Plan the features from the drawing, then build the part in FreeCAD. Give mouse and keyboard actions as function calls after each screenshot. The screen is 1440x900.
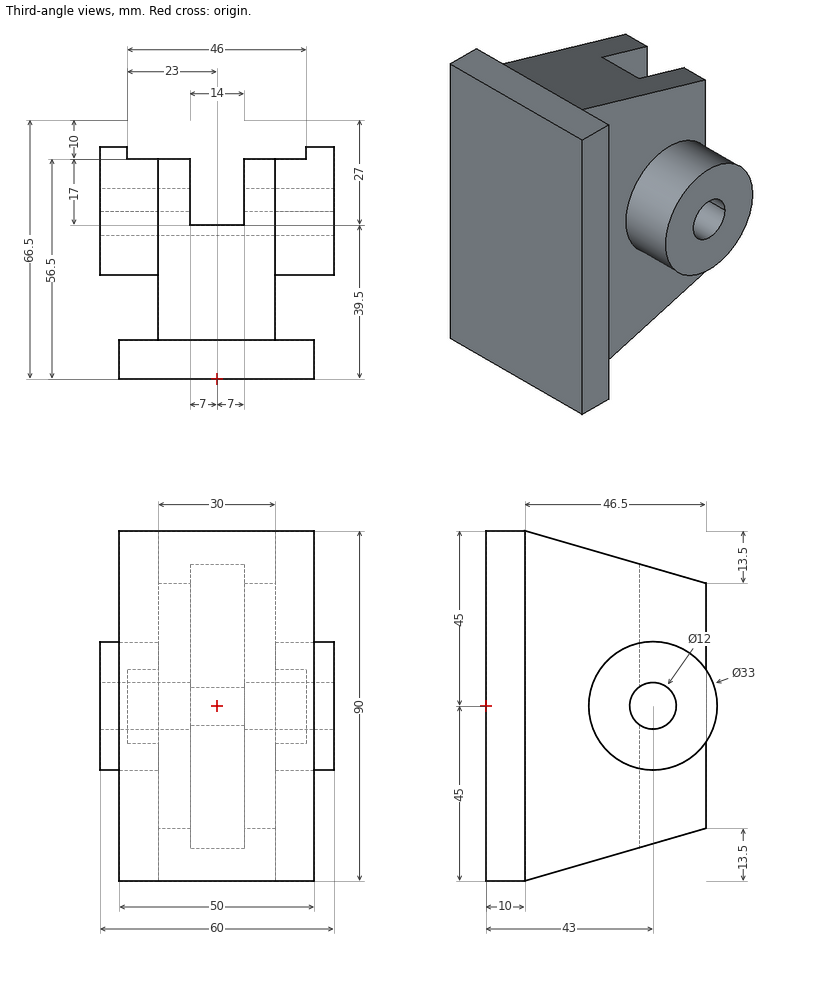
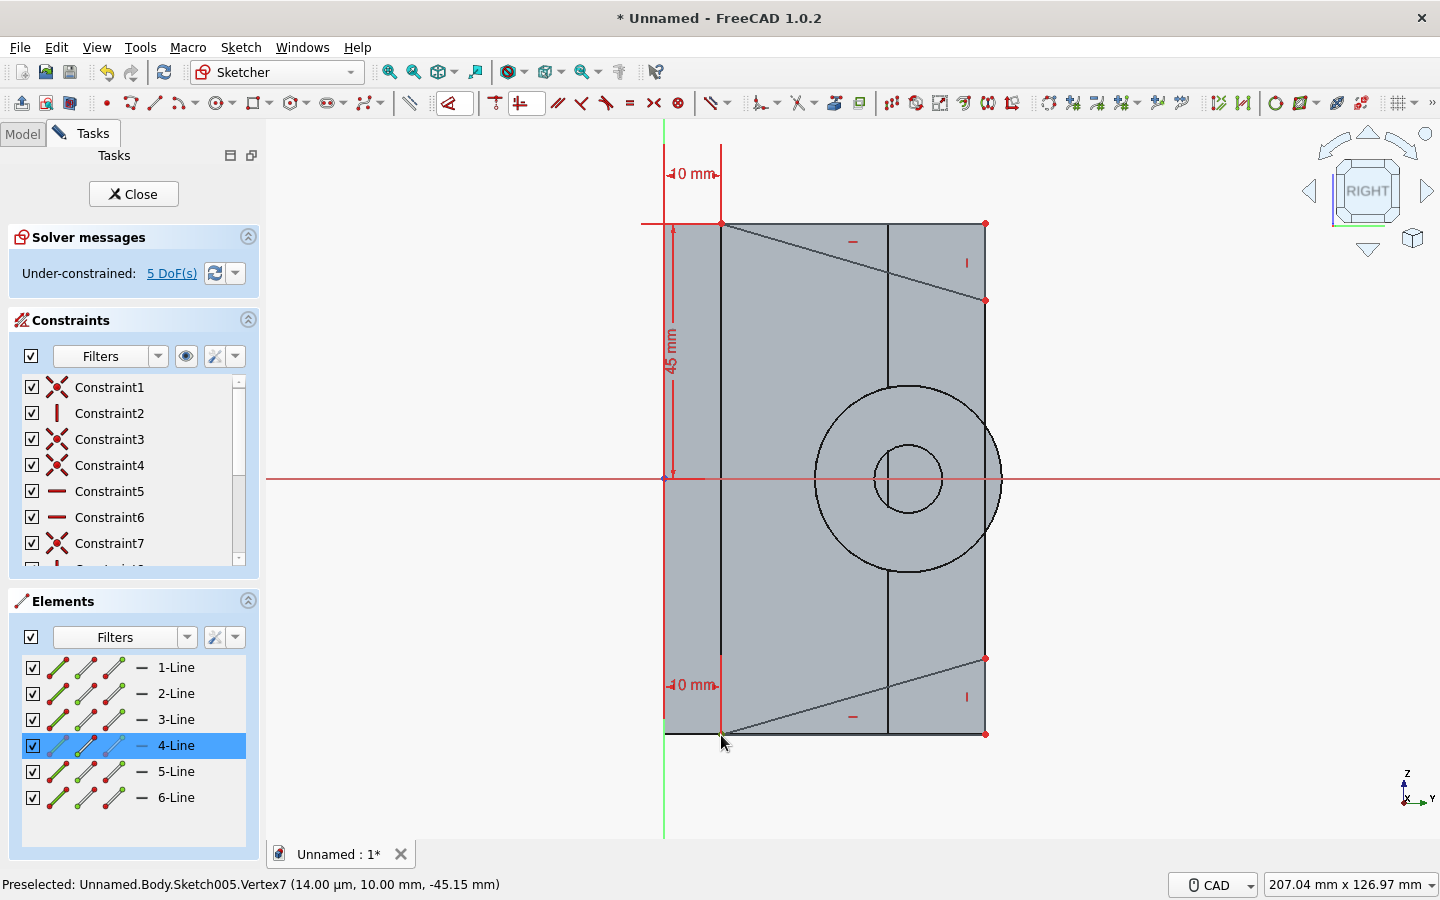
click(468, 104)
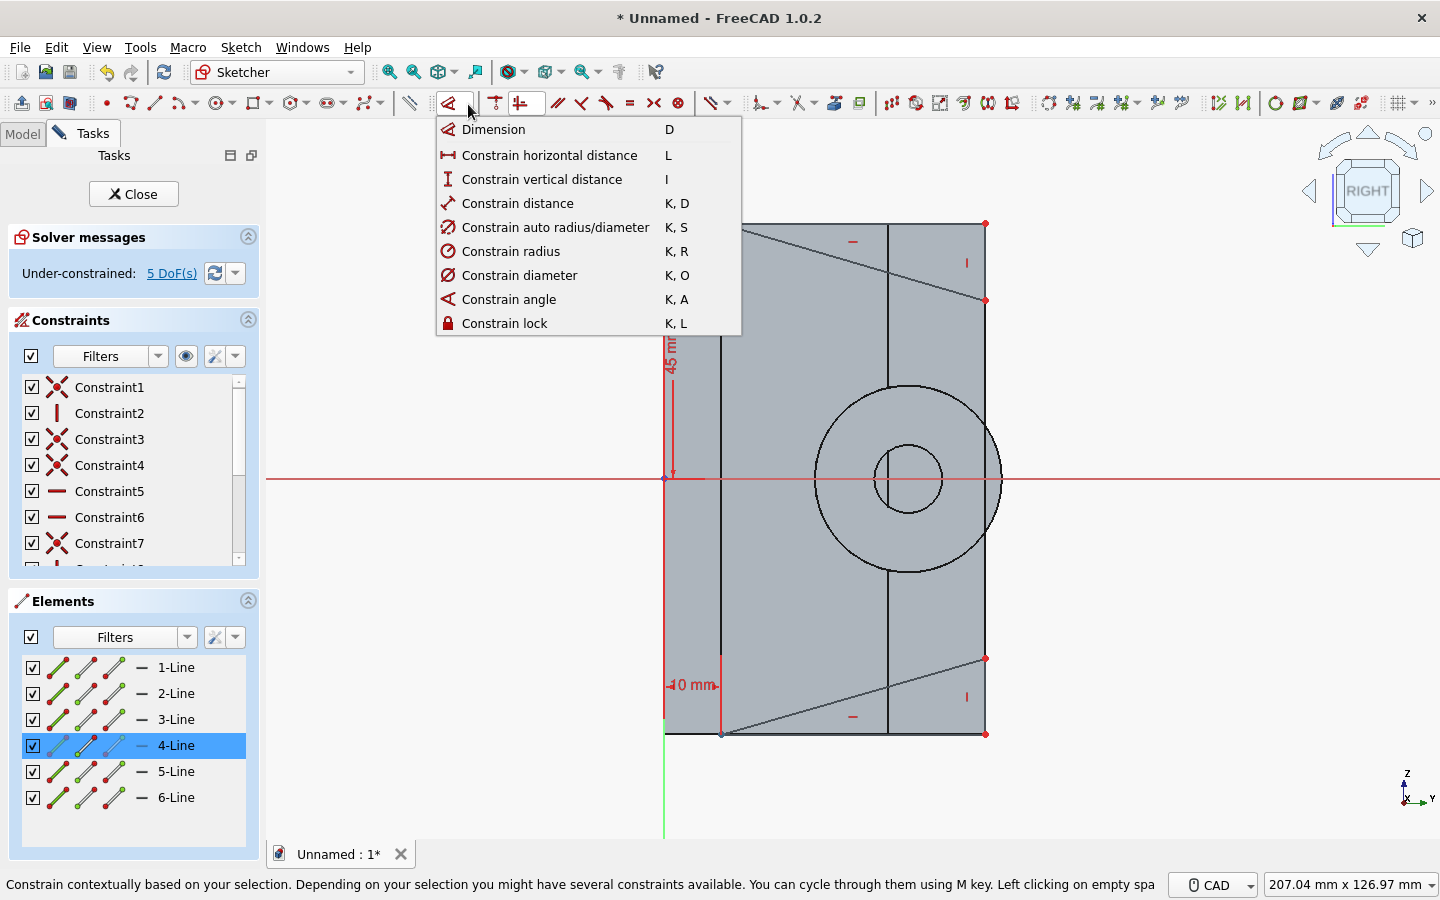
click(589, 179)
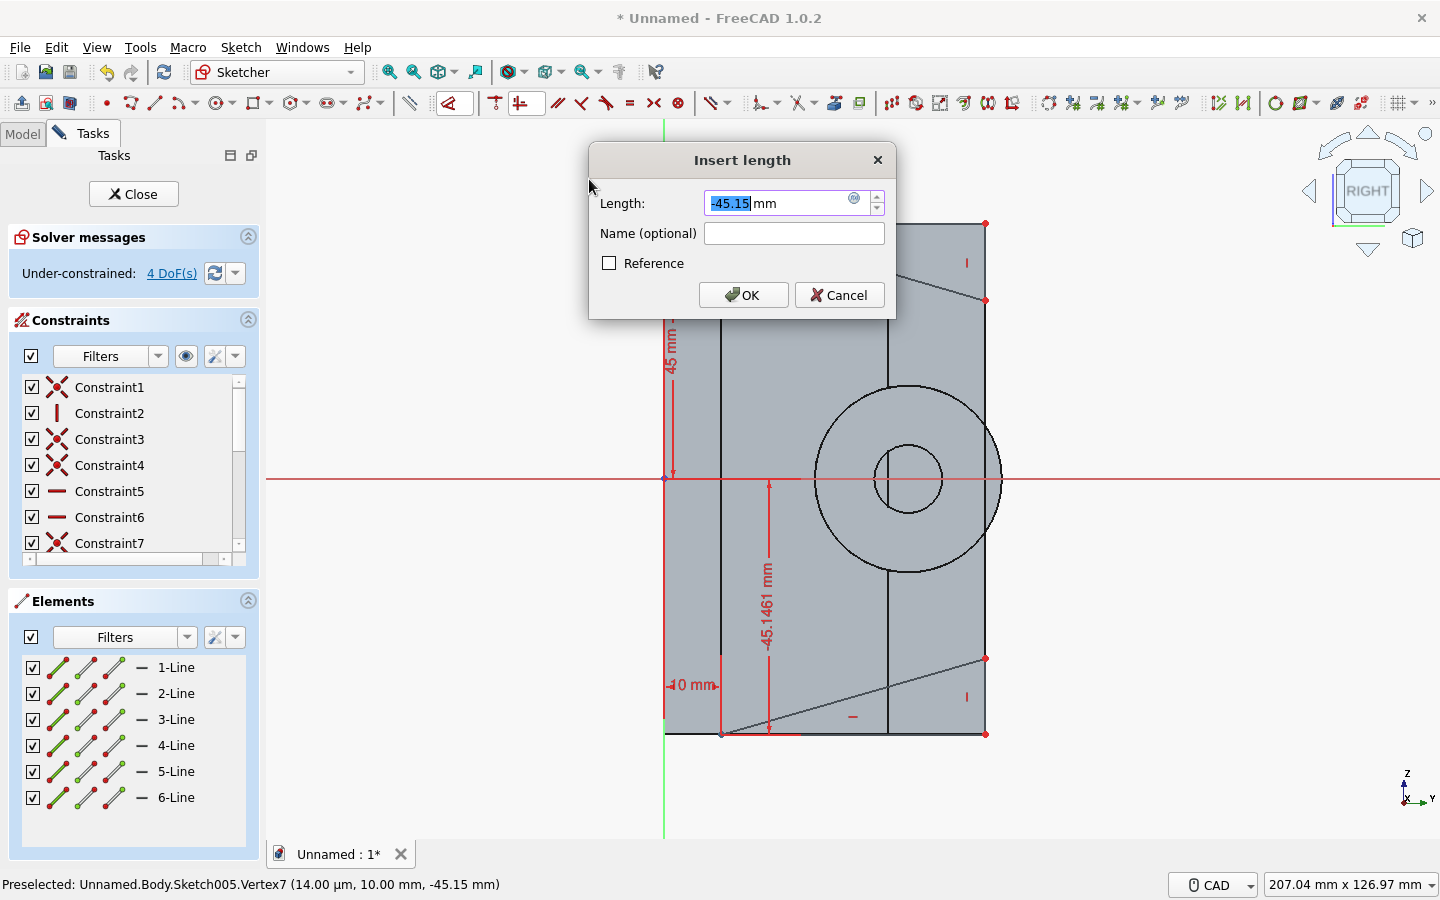
text(-45)
key(Return)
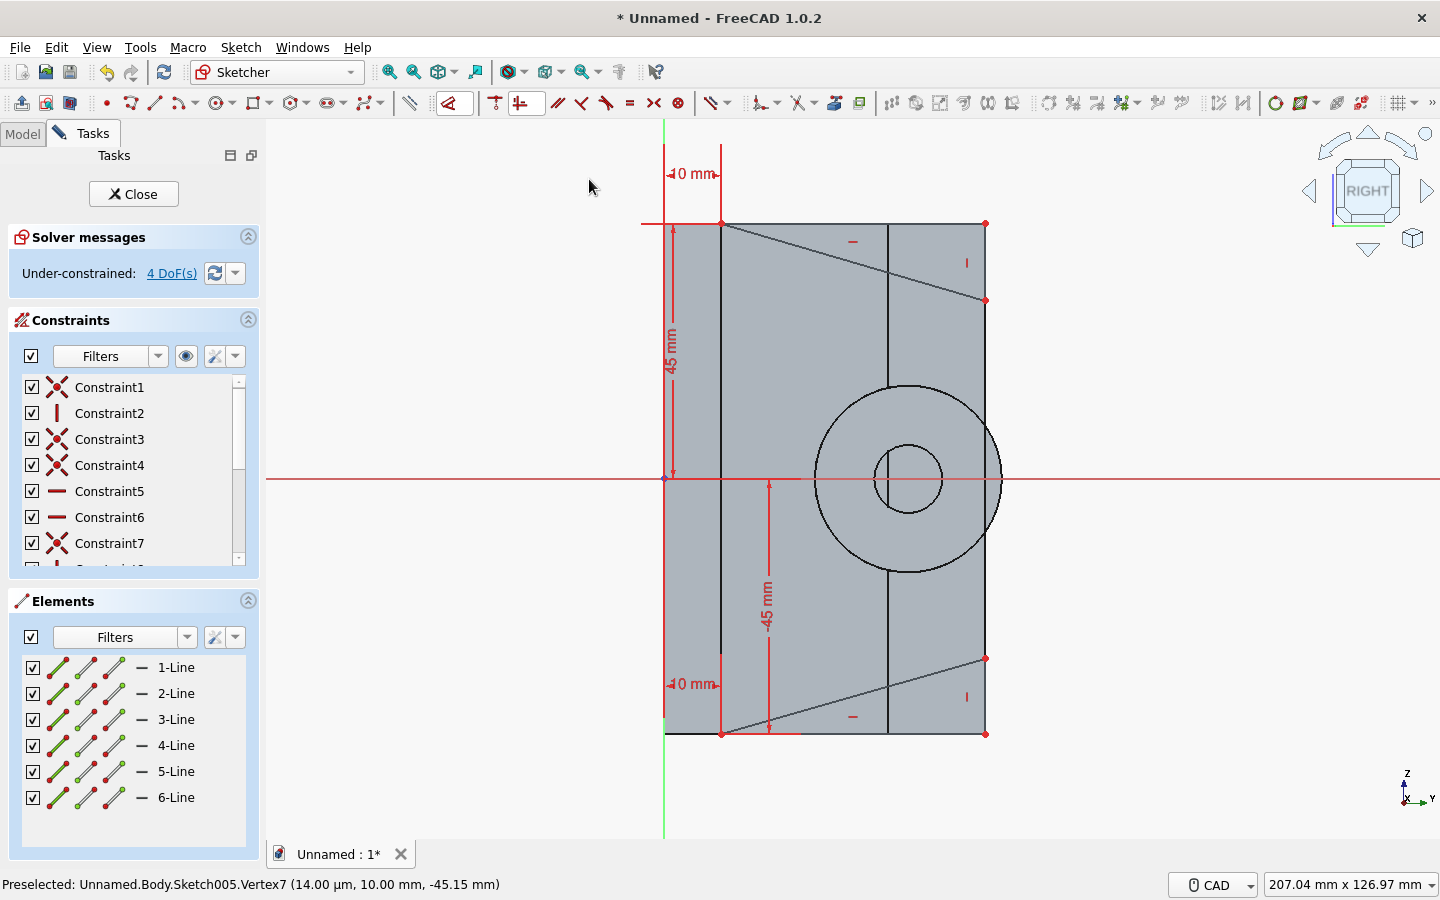
click(985, 278)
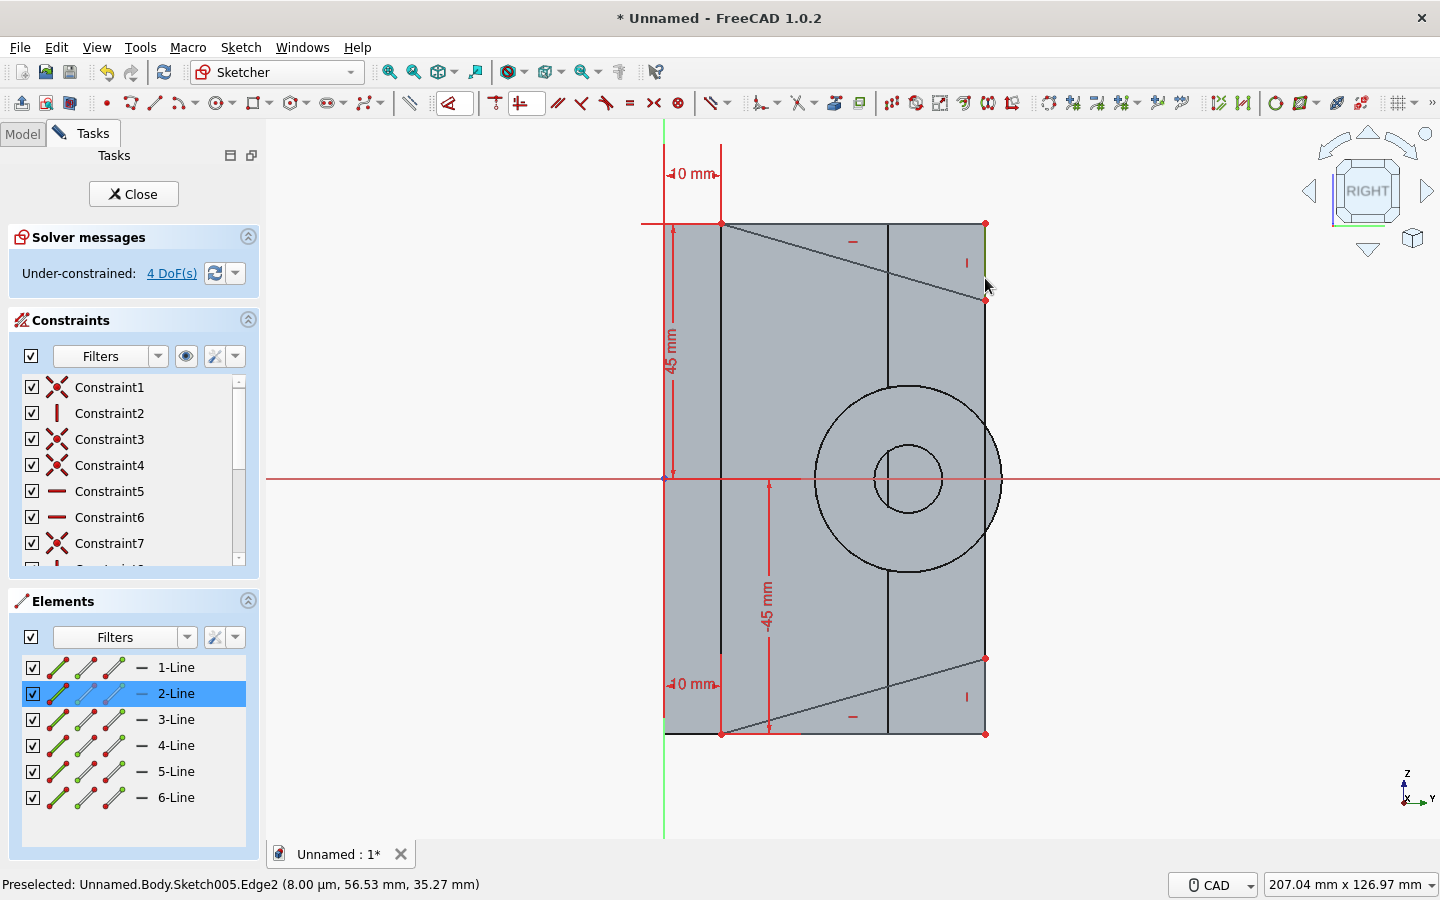
click(468, 104)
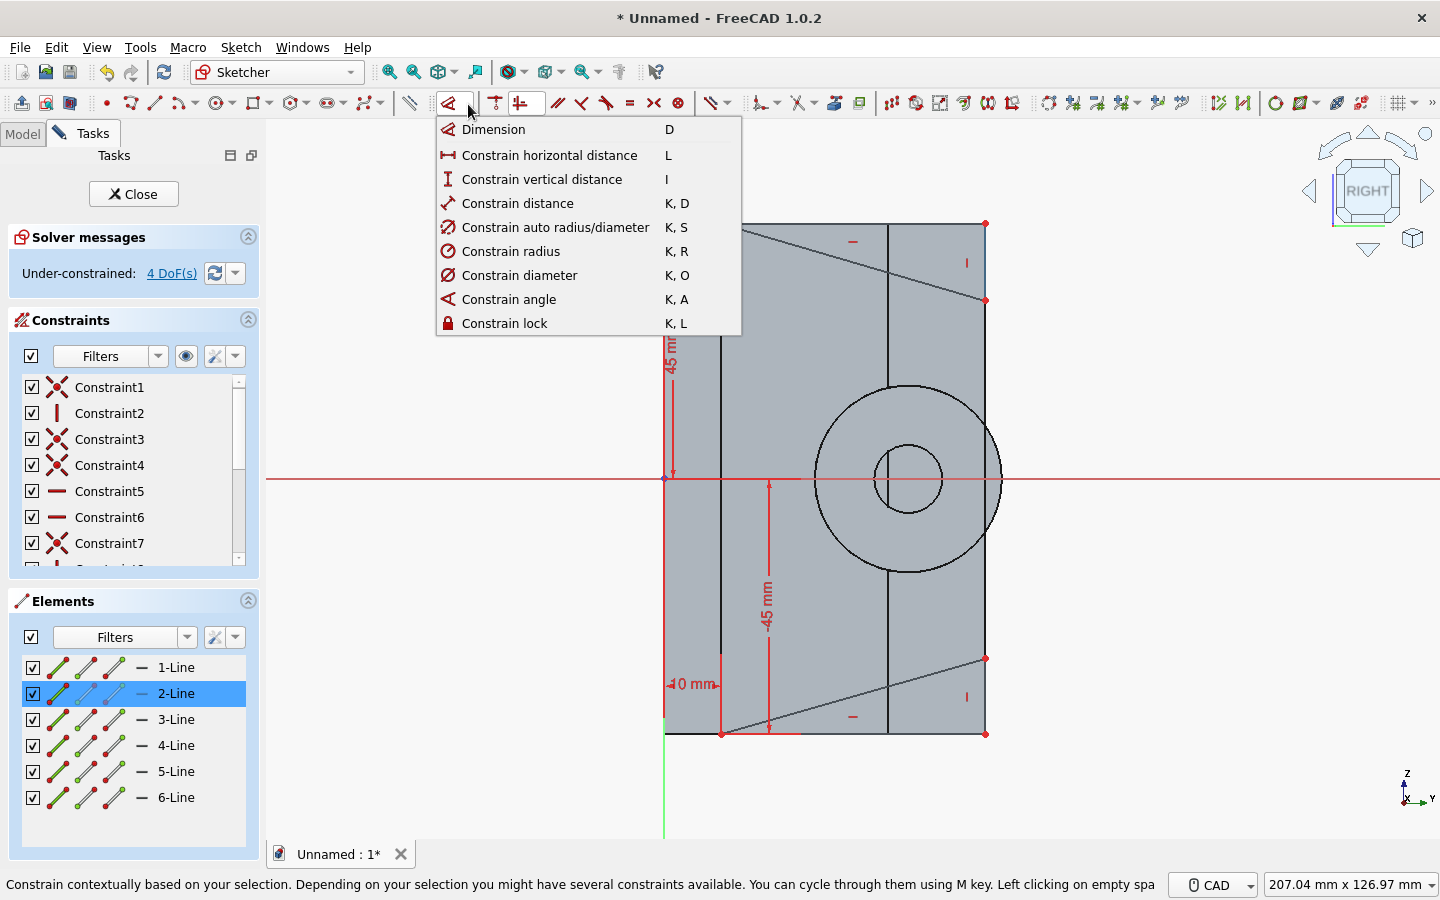
click(589, 179)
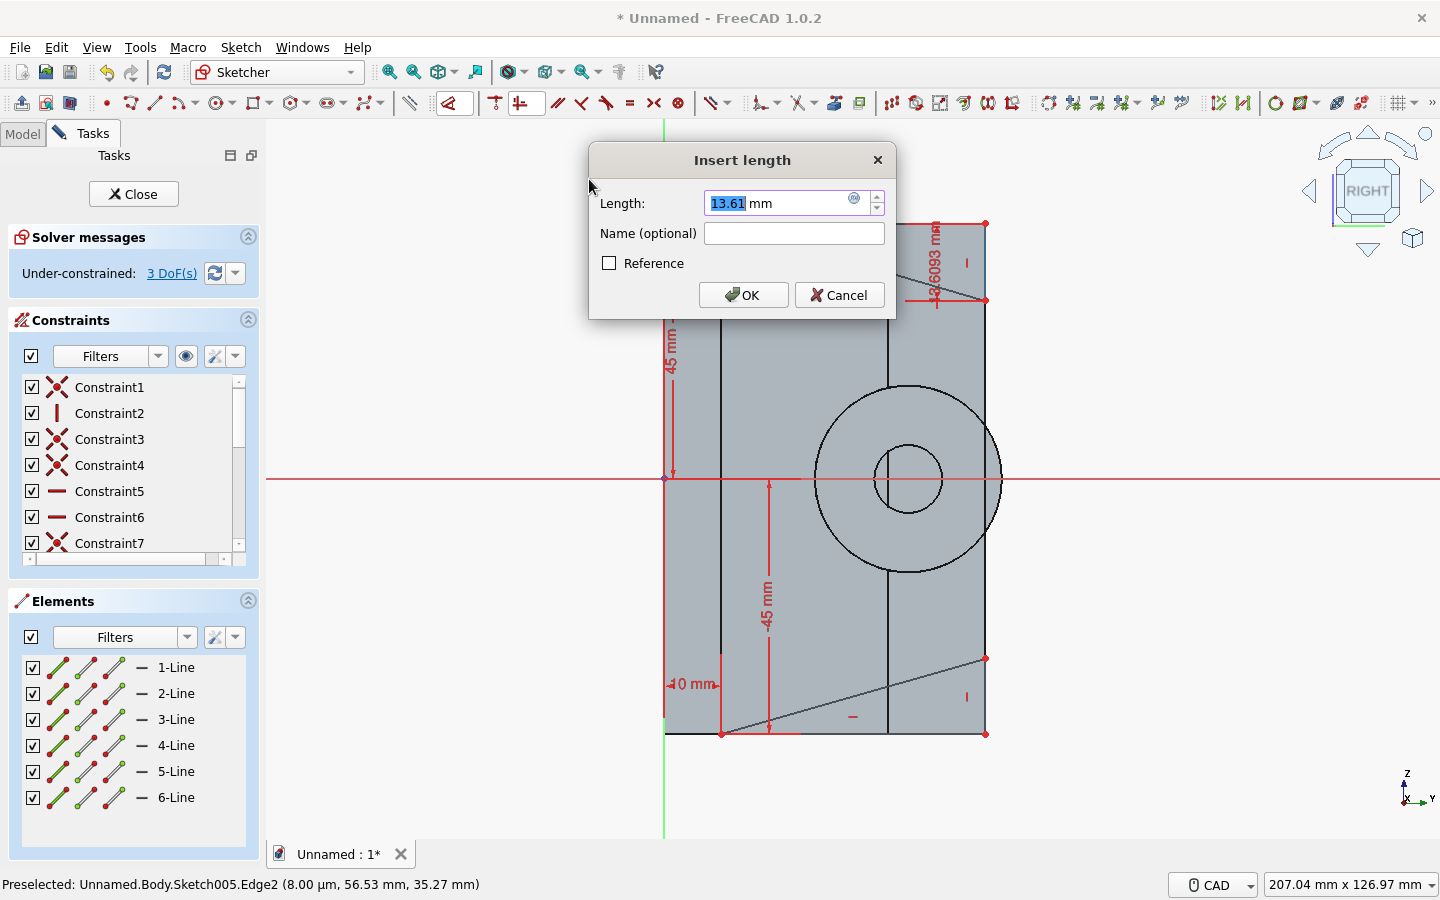
text(13.5)
key(Return)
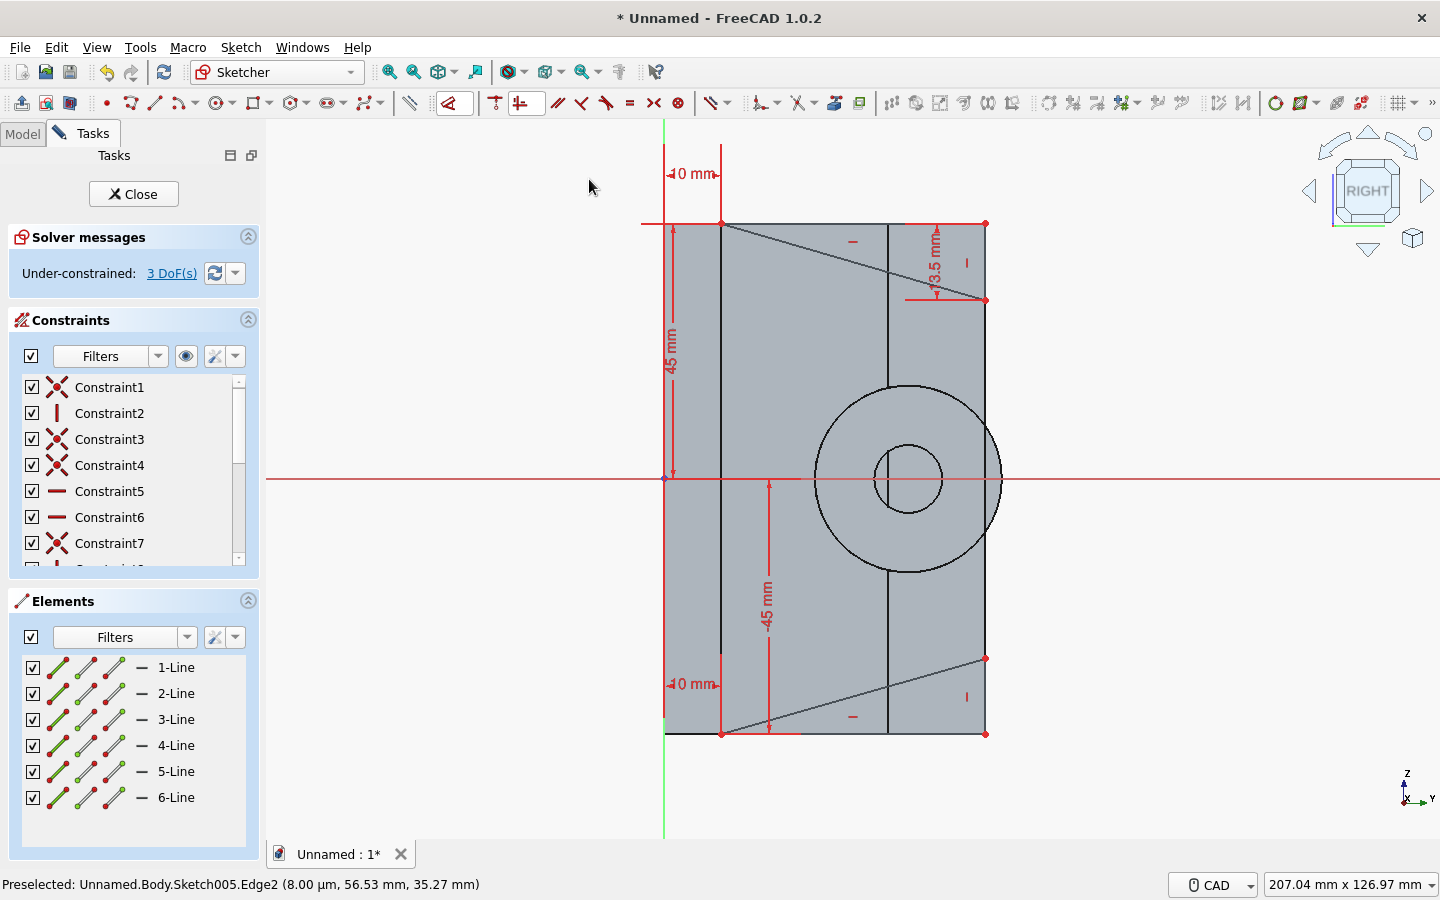
click(906, 224)